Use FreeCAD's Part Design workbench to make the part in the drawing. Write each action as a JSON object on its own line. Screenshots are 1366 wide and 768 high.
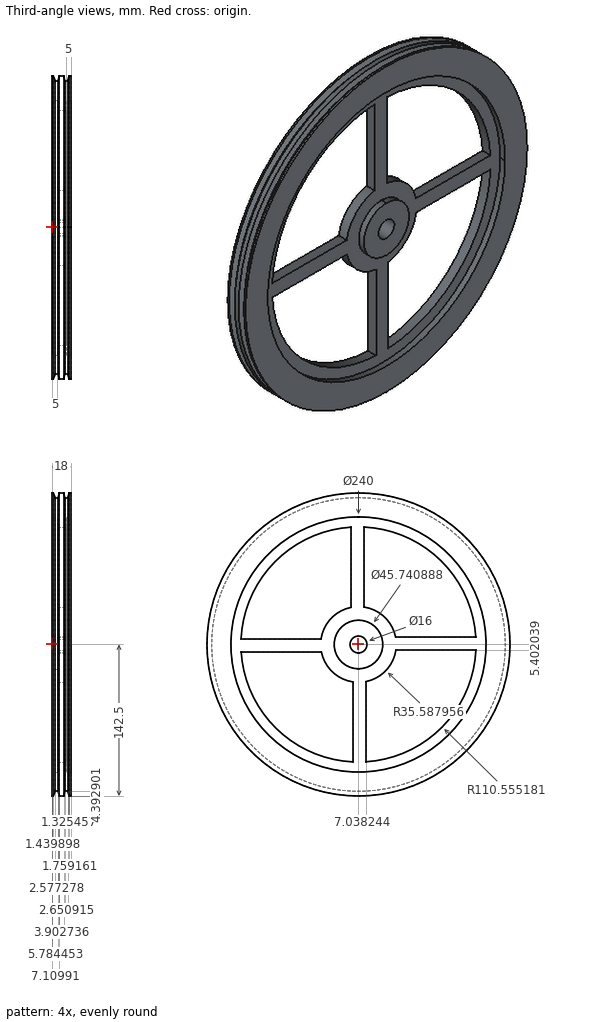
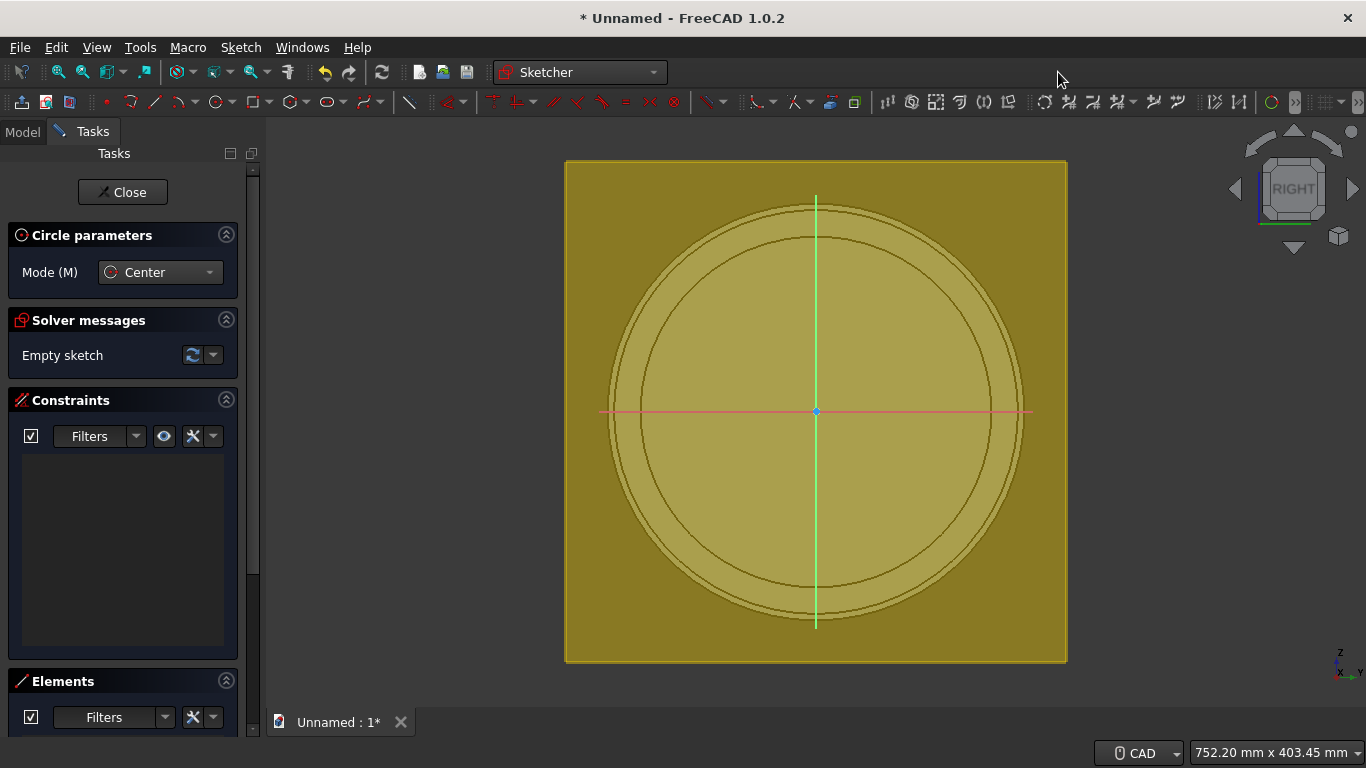
{"action": "left_click", "coordinate": [816, 412]}
{"action": "mouse_move", "coordinate": [940, 288]}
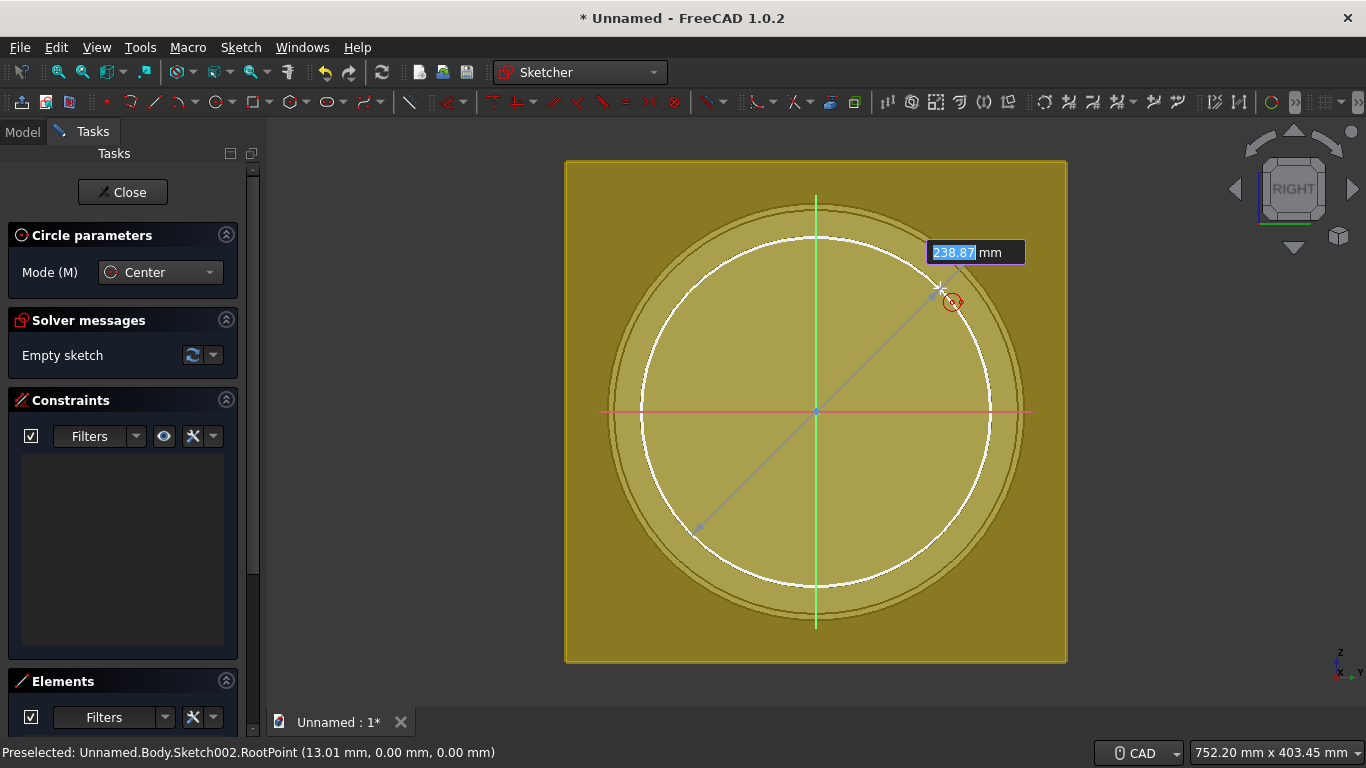
{"action": "type", "text": "240"}
{"action": "key", "text": "Return"}
{"action": "key", "text": "Escape"}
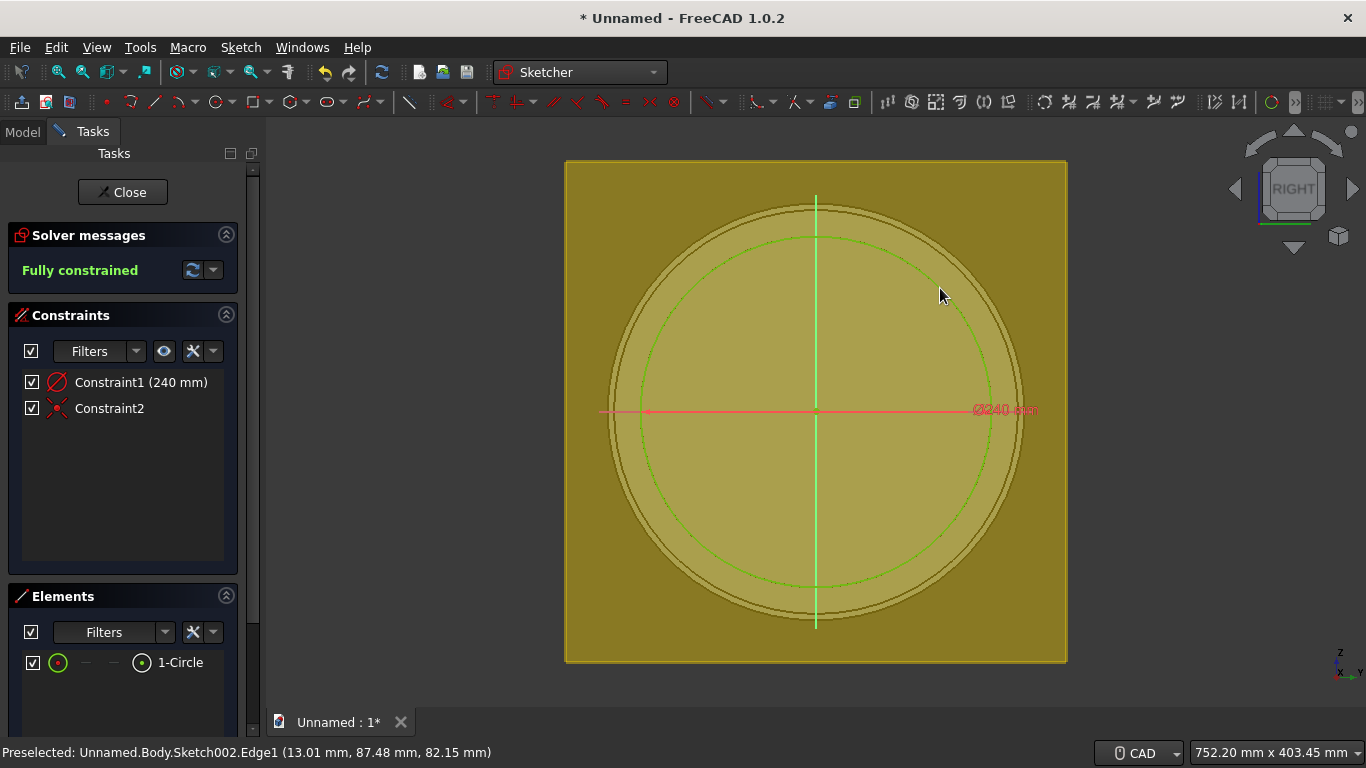
{"action": "left_click", "coordinate": [123, 192]}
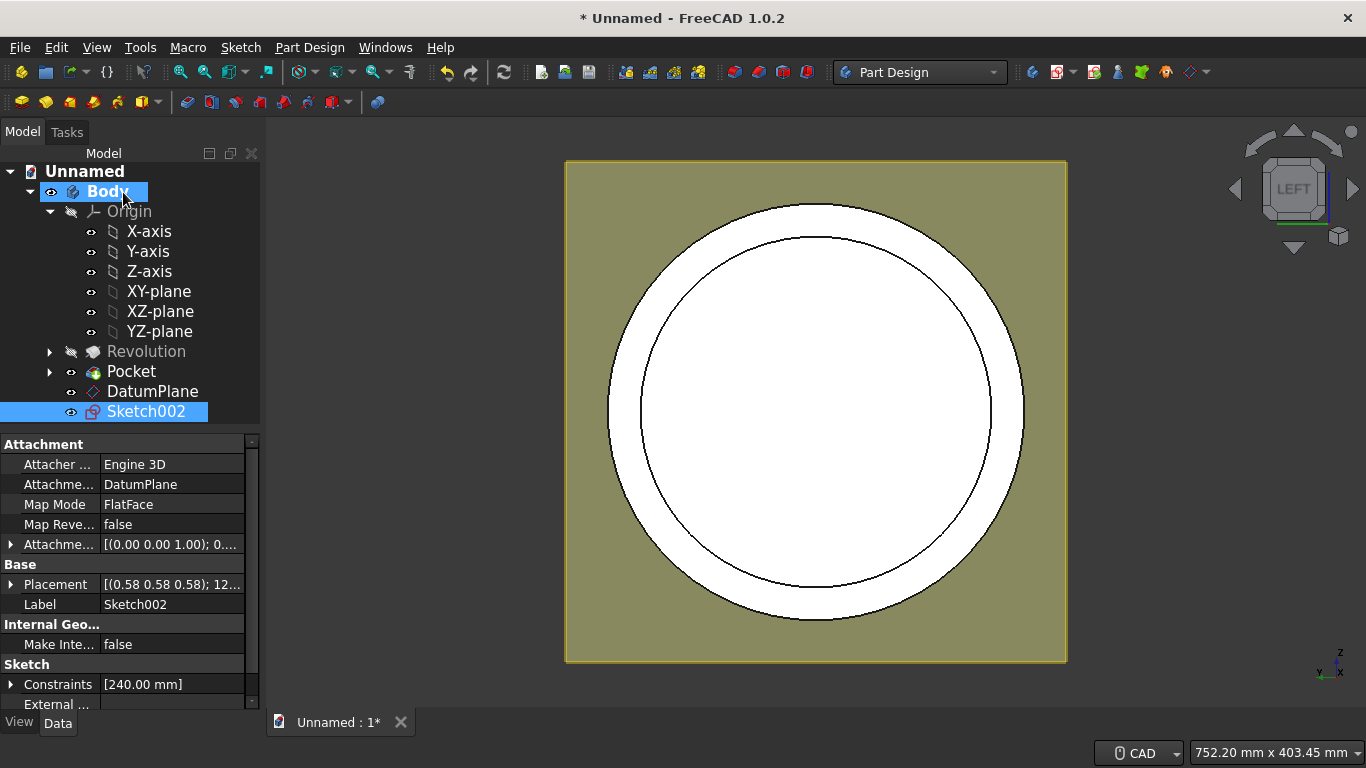
{"action": "left_click", "coordinate": [188, 102]}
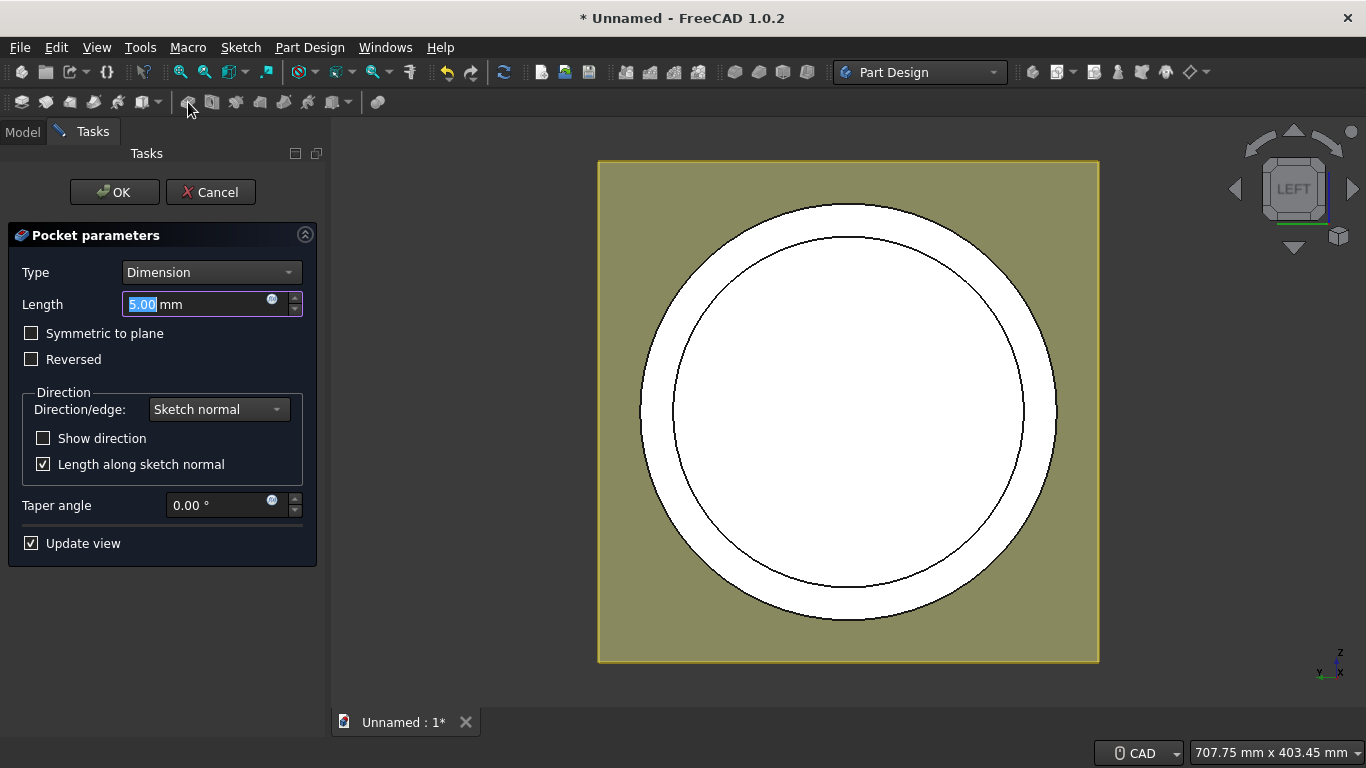
{"action": "type", "text": "5"}
{"action": "key", "text": "Tab"}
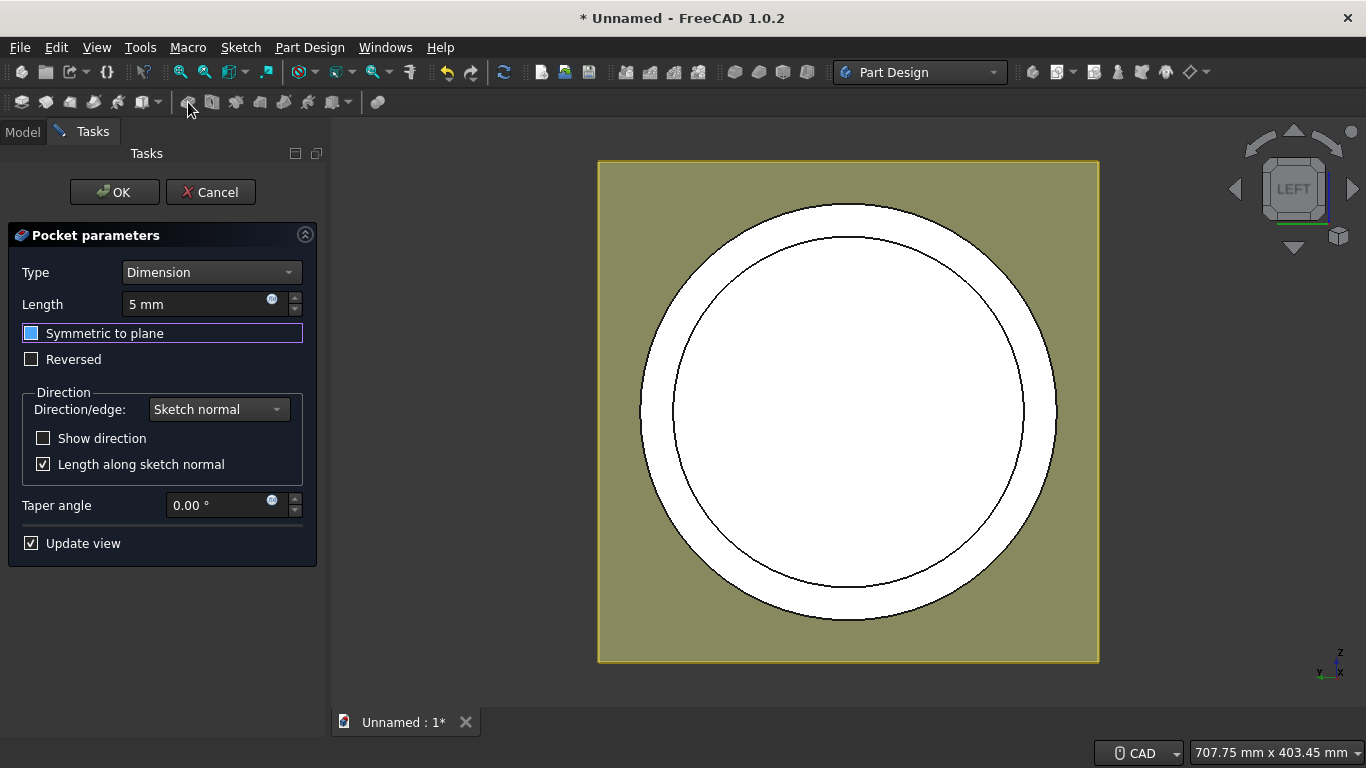
{"action": "left_click", "coordinate": [30, 359]}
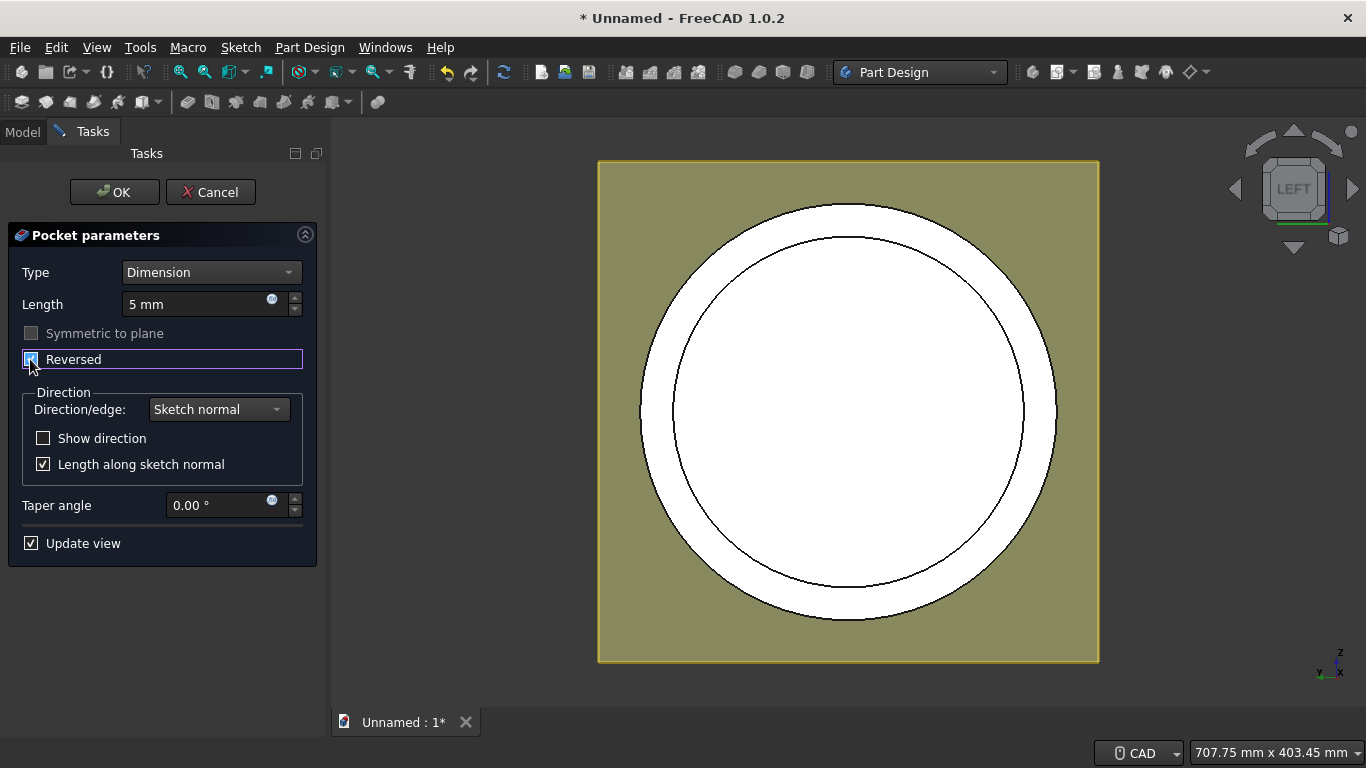
{"action": "left_click", "coordinate": [115, 192]}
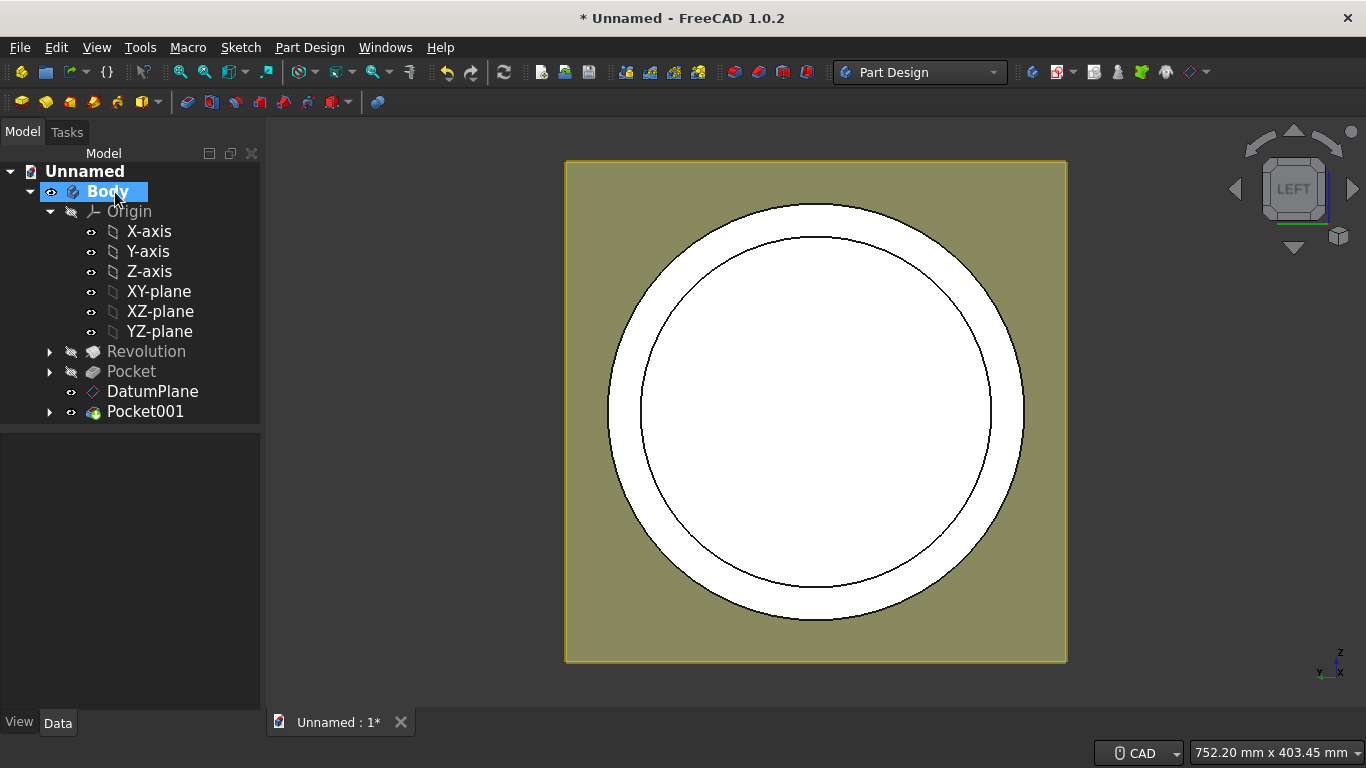
{"action": "left_click", "coordinate": [116, 392]}
{"action": "key", "text": "space"}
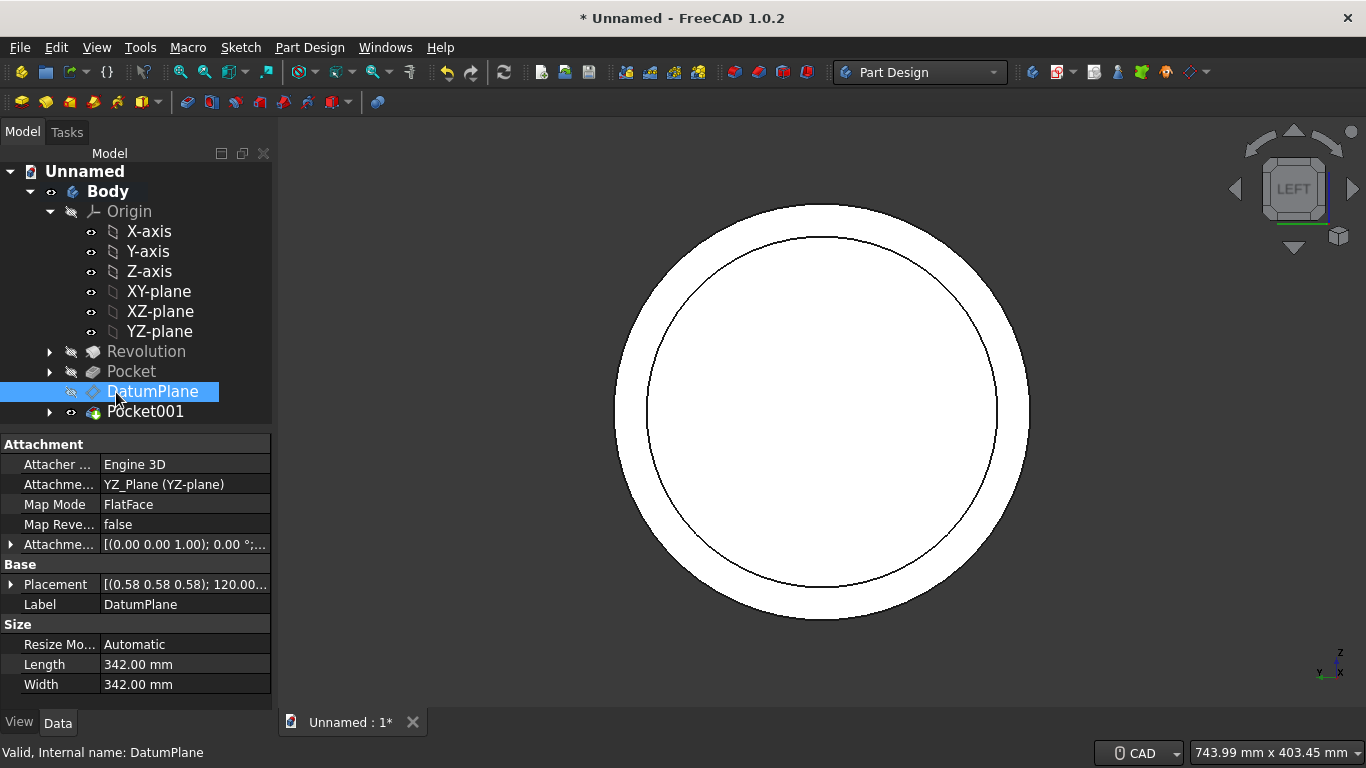
{"action": "key", "text": "0"}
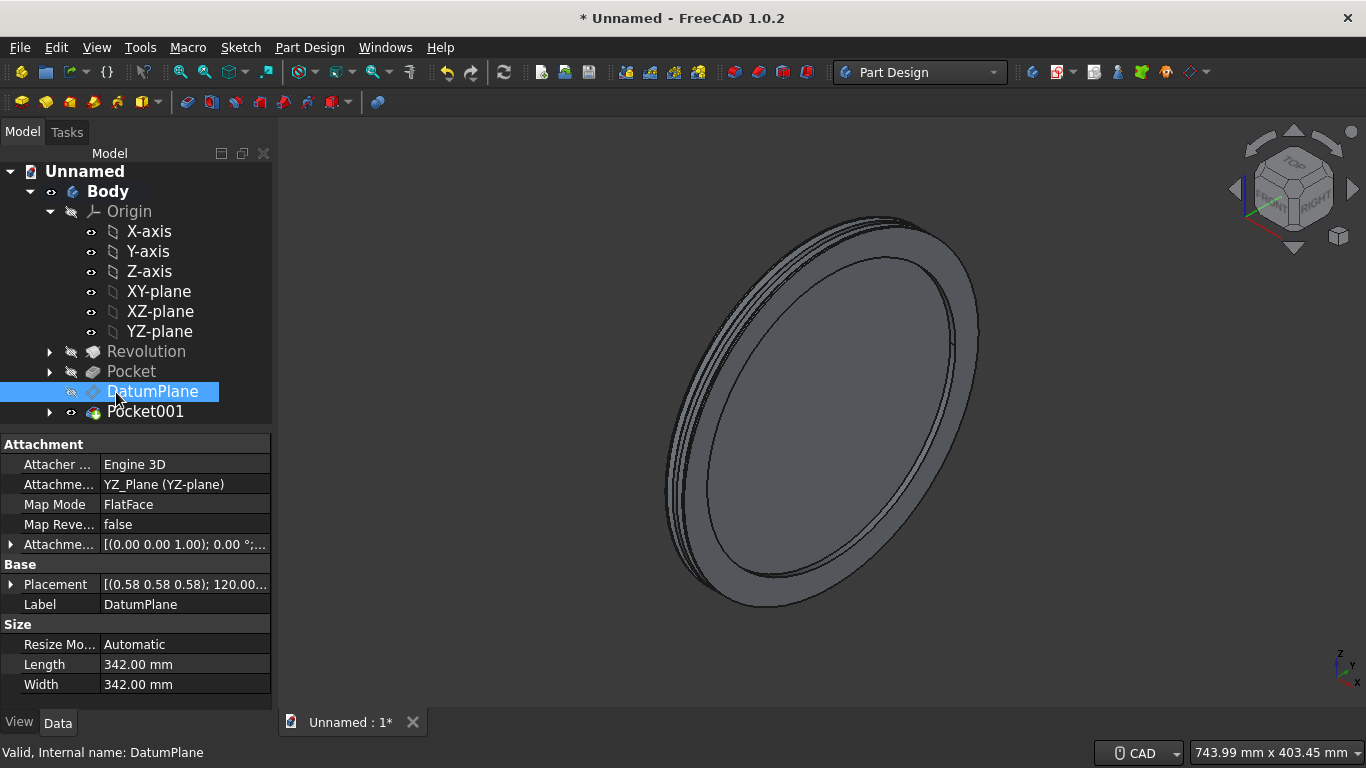
{"action": "left_click", "coordinate": [826, 413]}